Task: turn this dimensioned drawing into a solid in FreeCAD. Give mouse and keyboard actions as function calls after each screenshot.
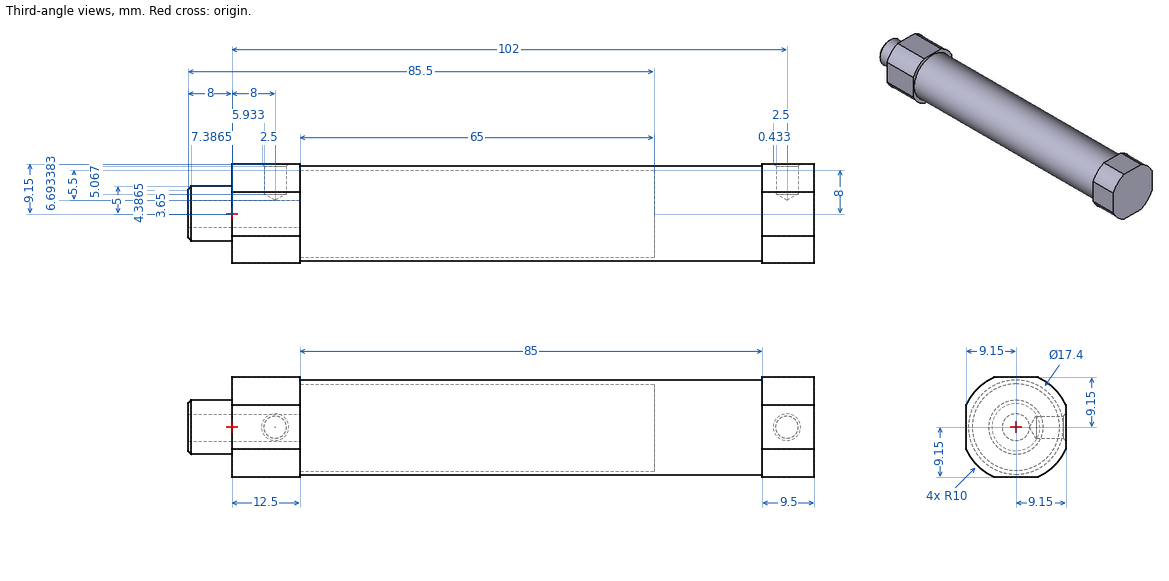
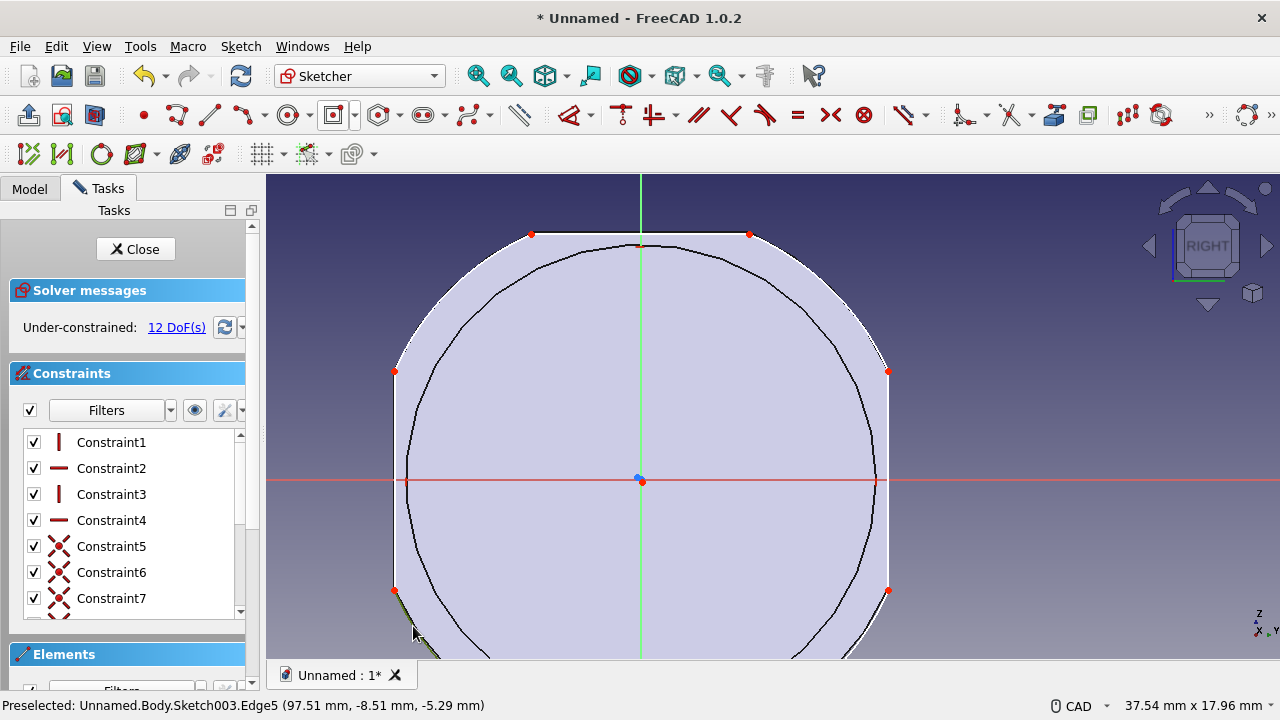
click(480, 264)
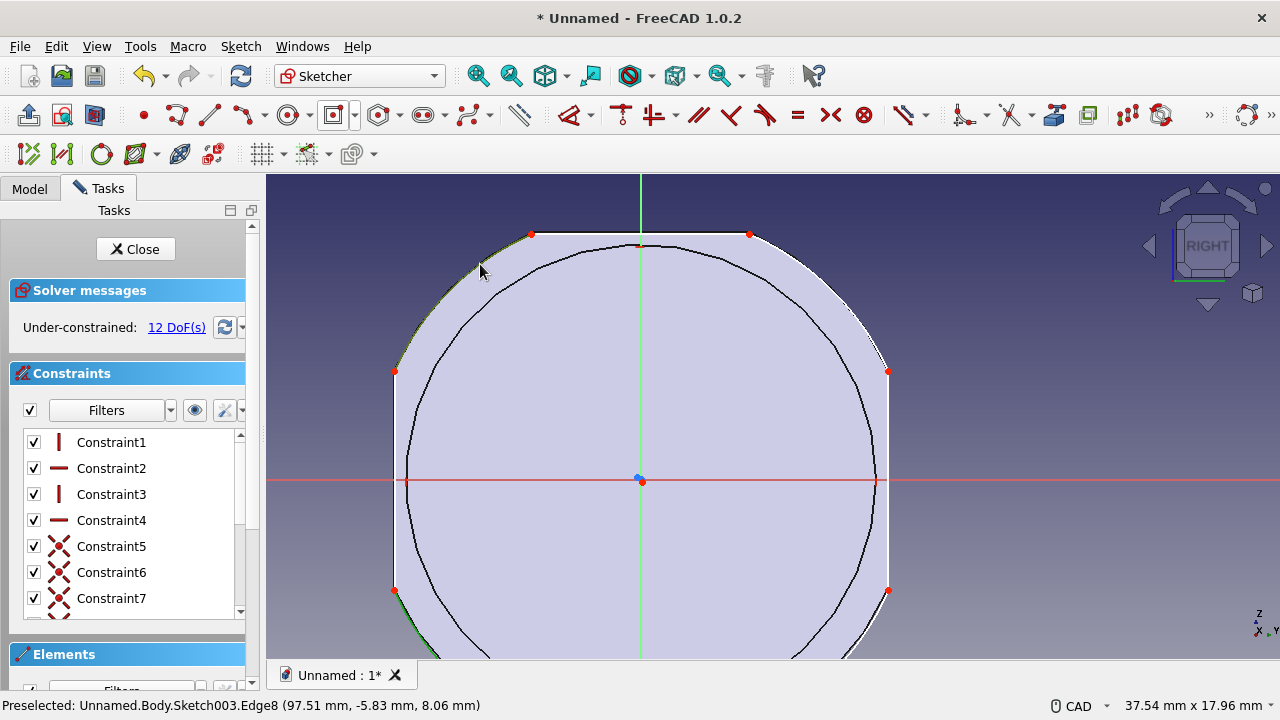
click(621, 116)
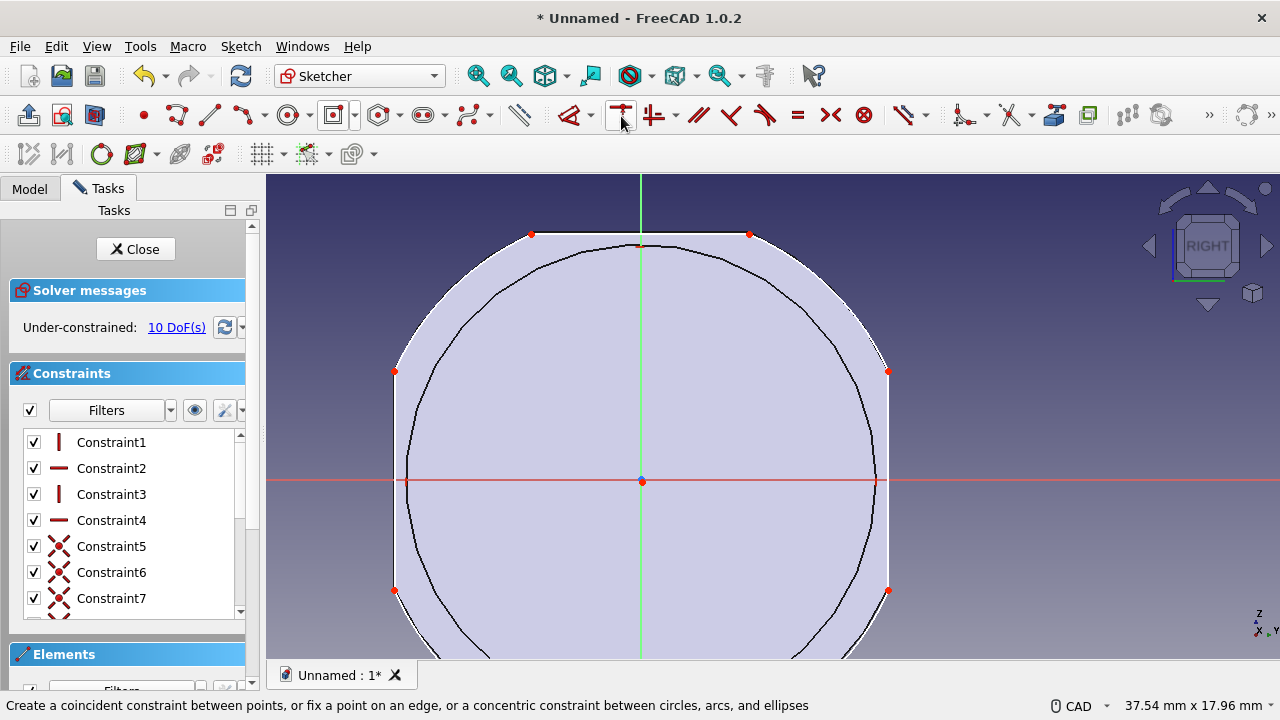
drag(631, 470, 652, 492)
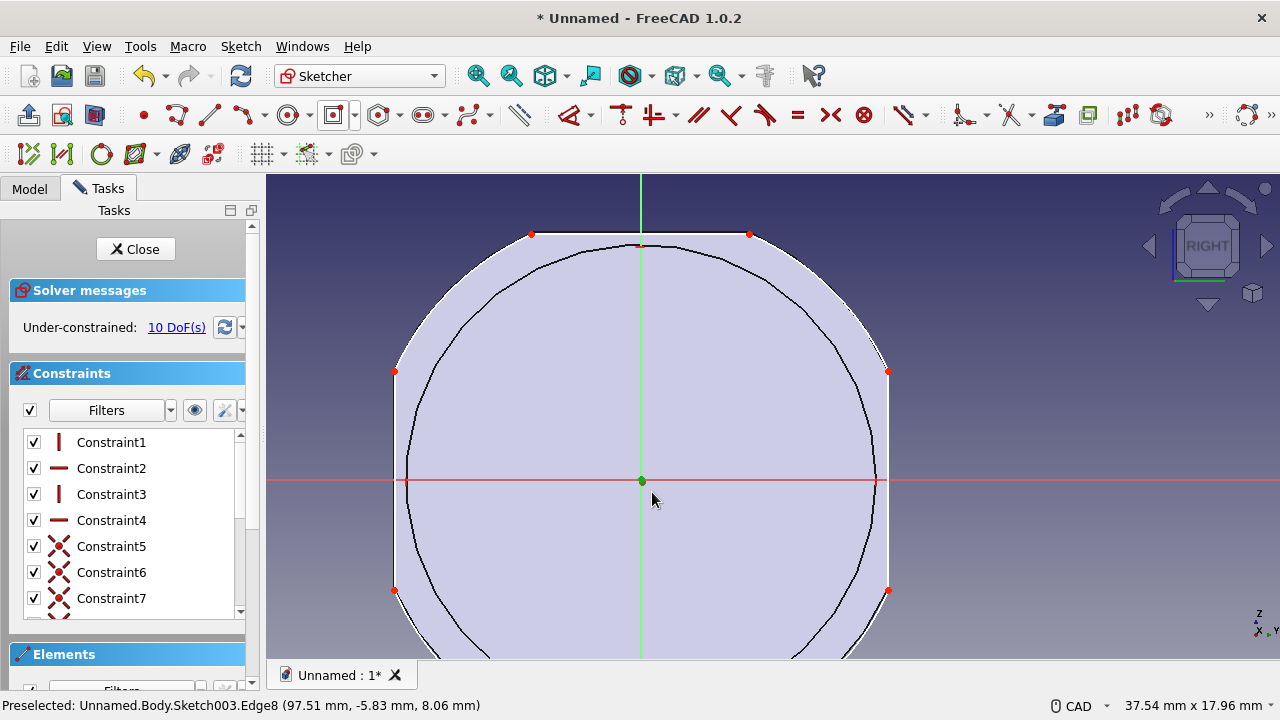
click(621, 116)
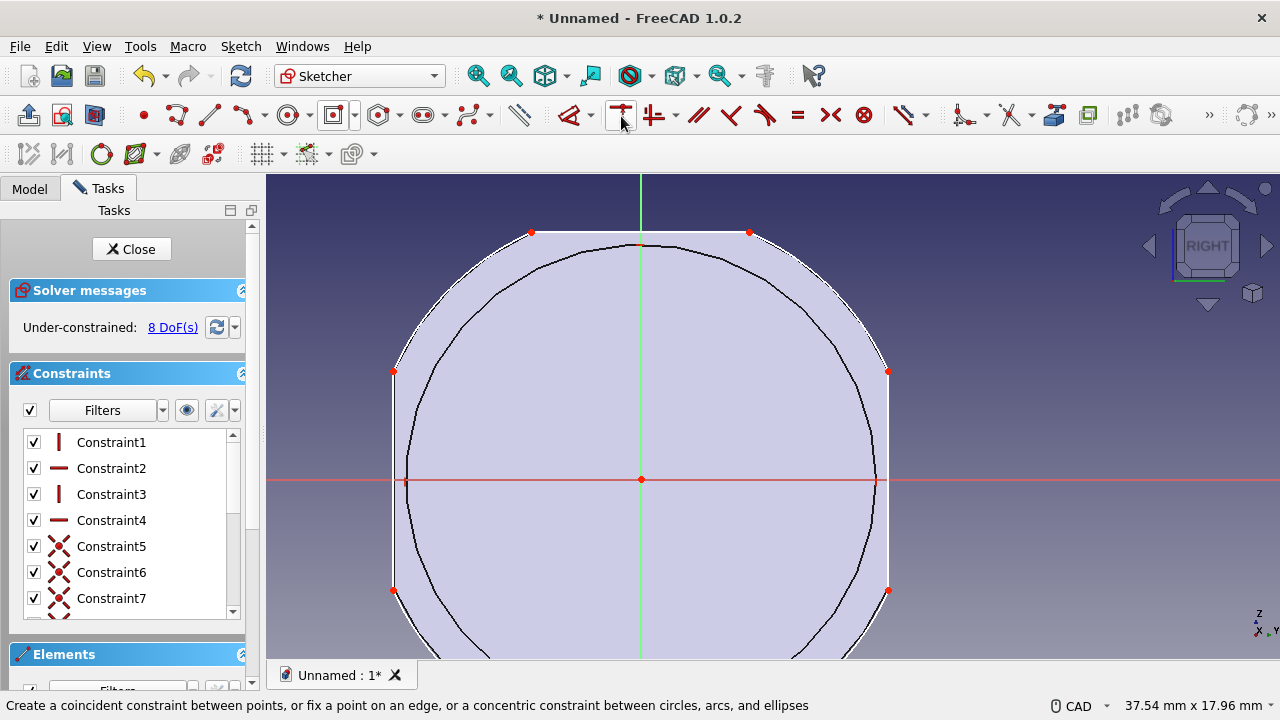
click(412, 626)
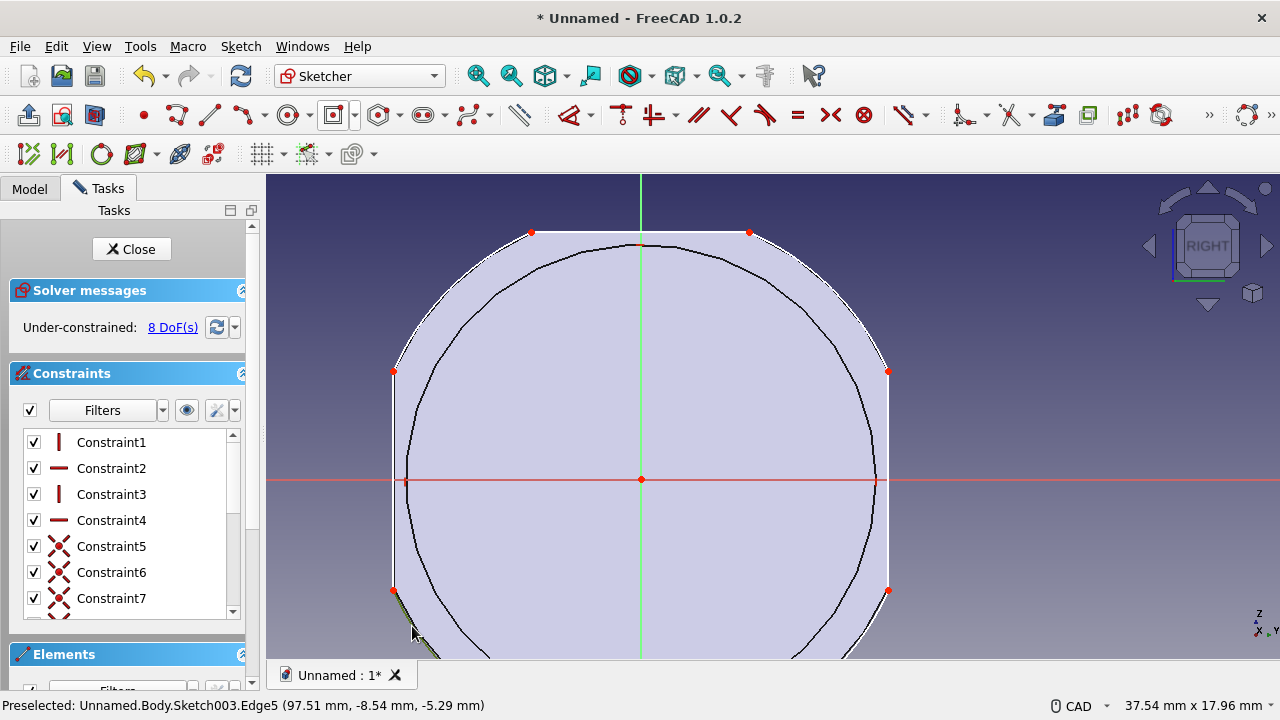
click(869, 626)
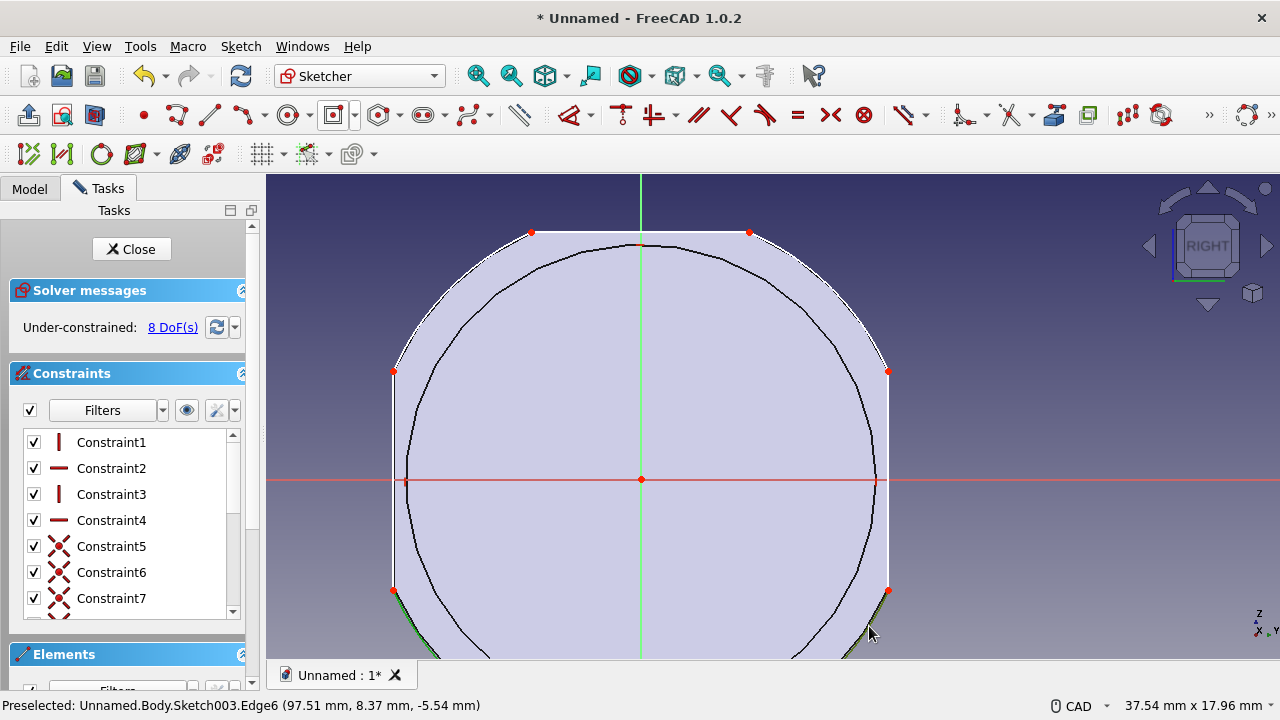
click(858, 319)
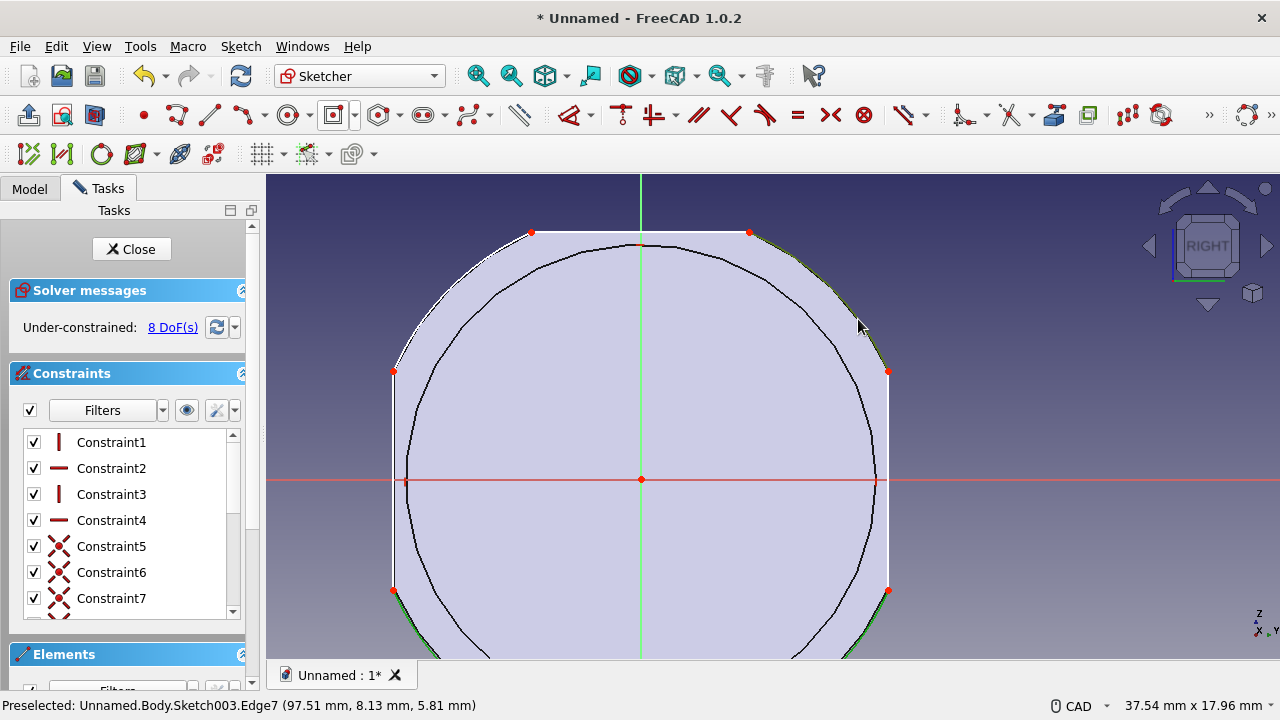
click(480, 263)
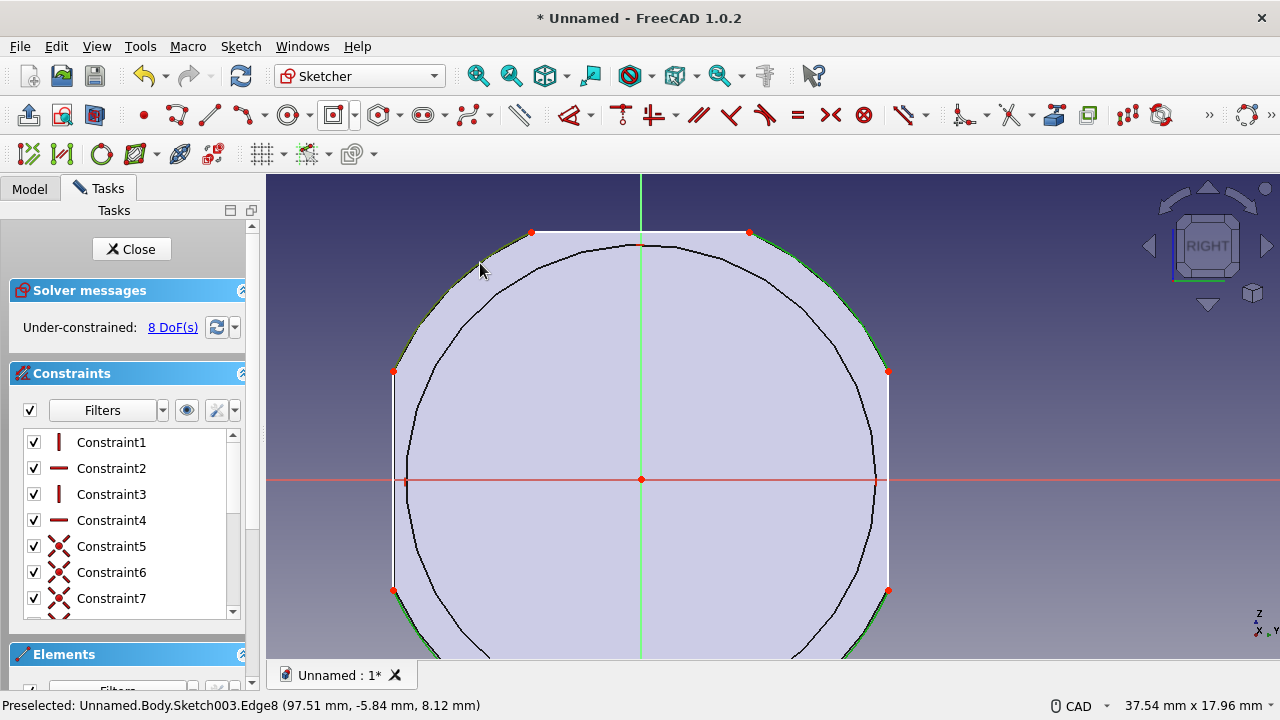
click(798, 116)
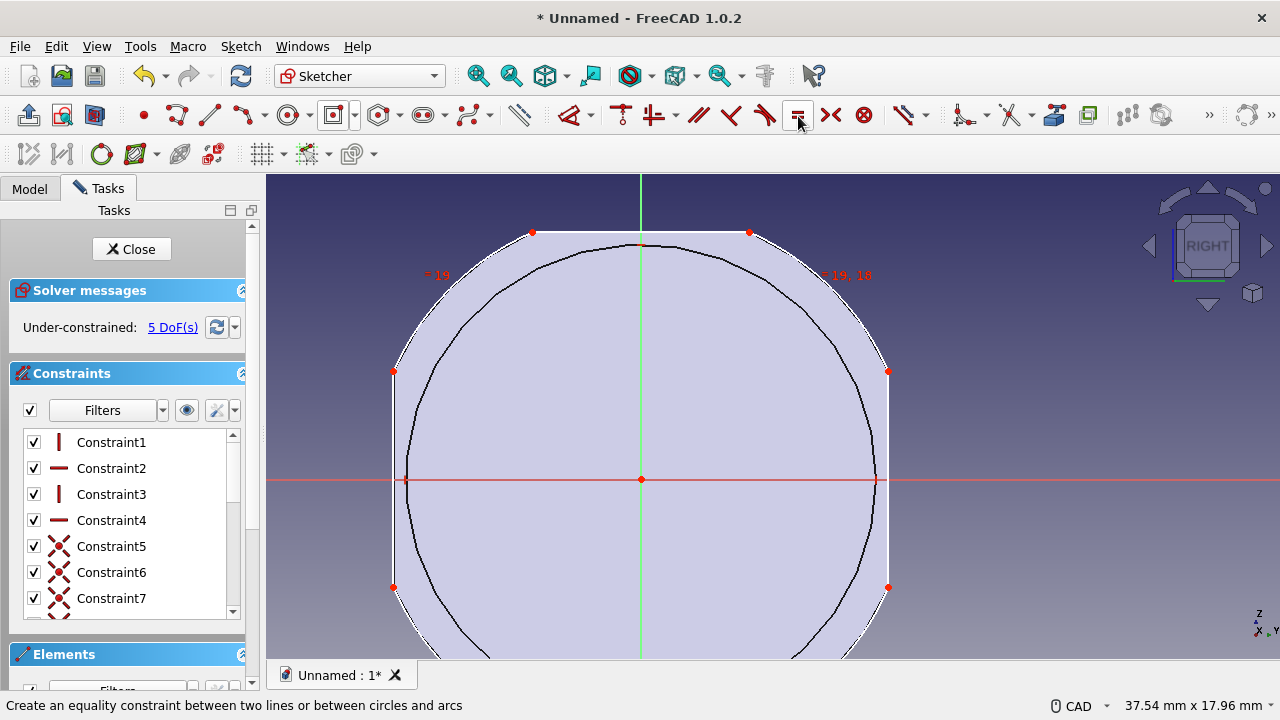
click(568, 116)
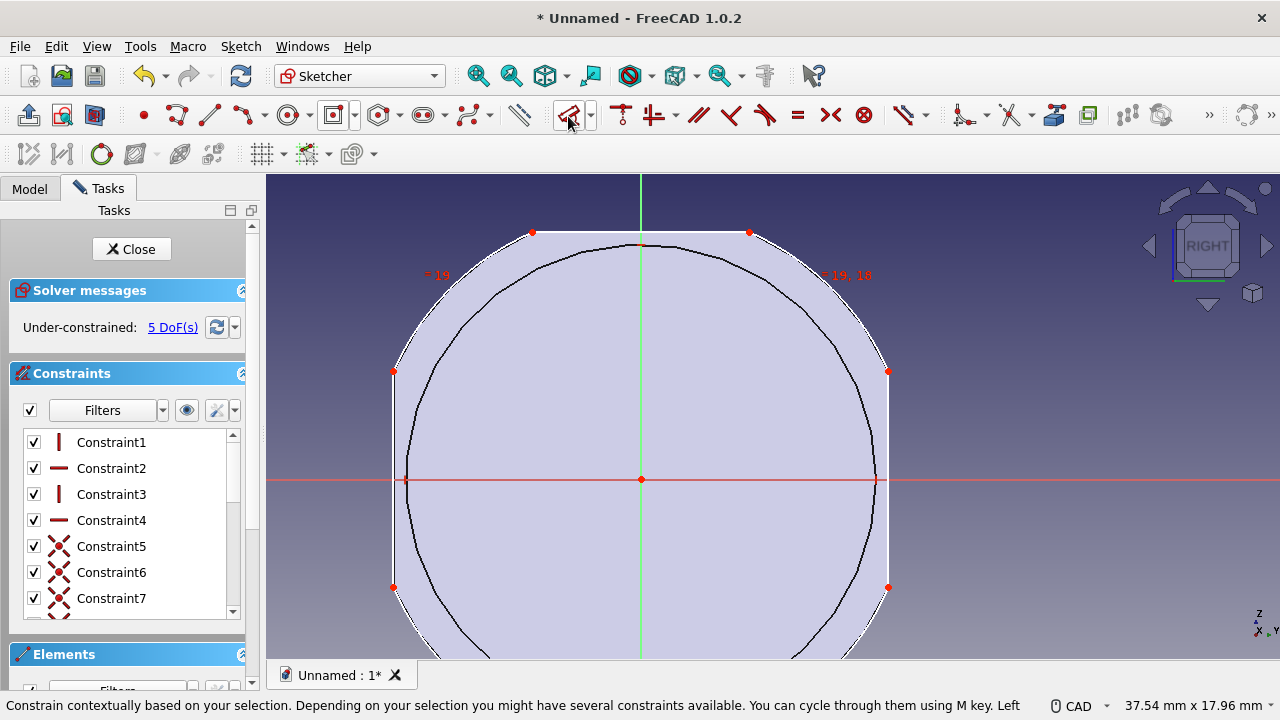
click(412, 623)
click(339, 498)